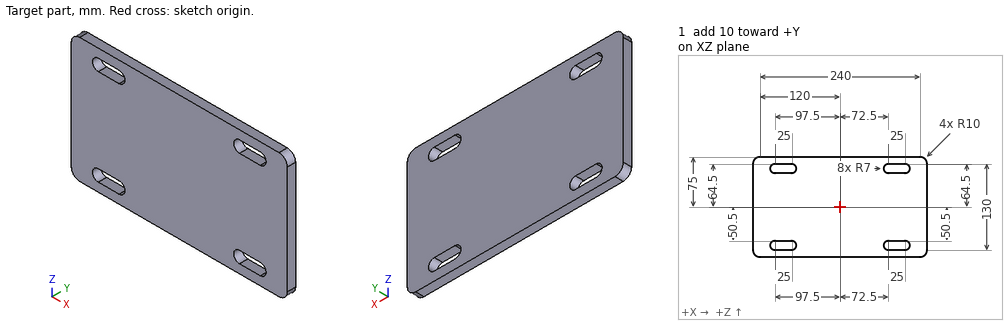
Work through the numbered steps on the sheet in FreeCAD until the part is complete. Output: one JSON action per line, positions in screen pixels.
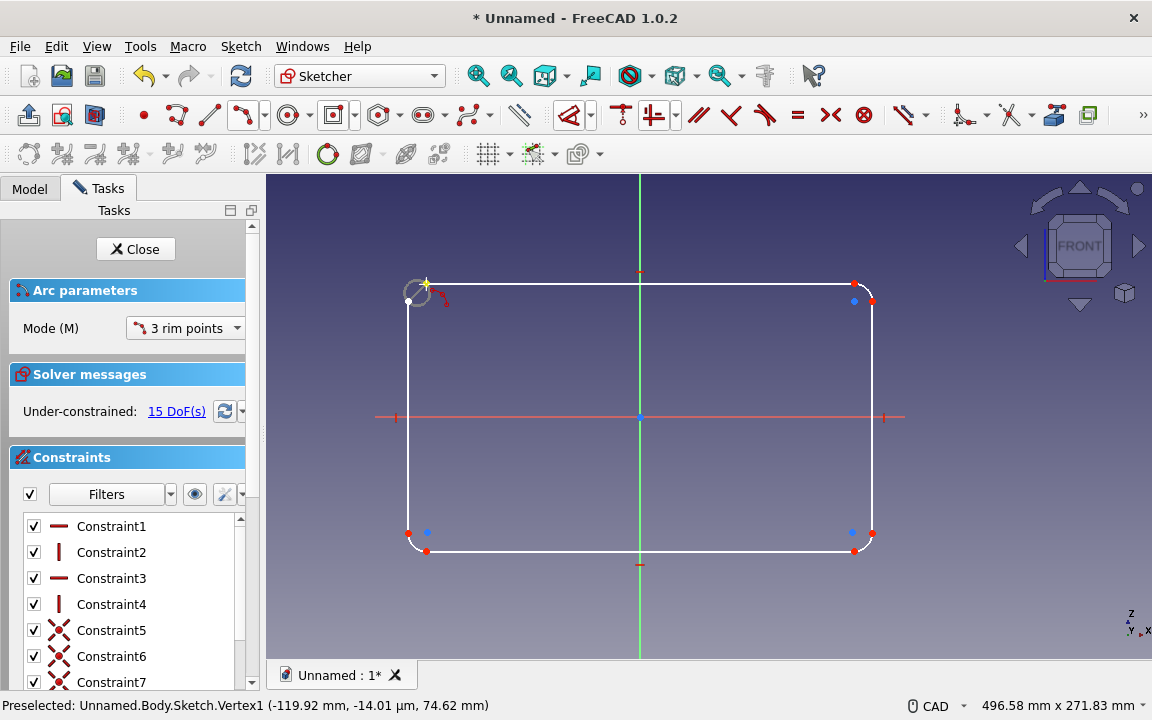
{"action": "scroll", "coordinate": [414, 289], "scroll_direction": "up", "scroll_amount": 6}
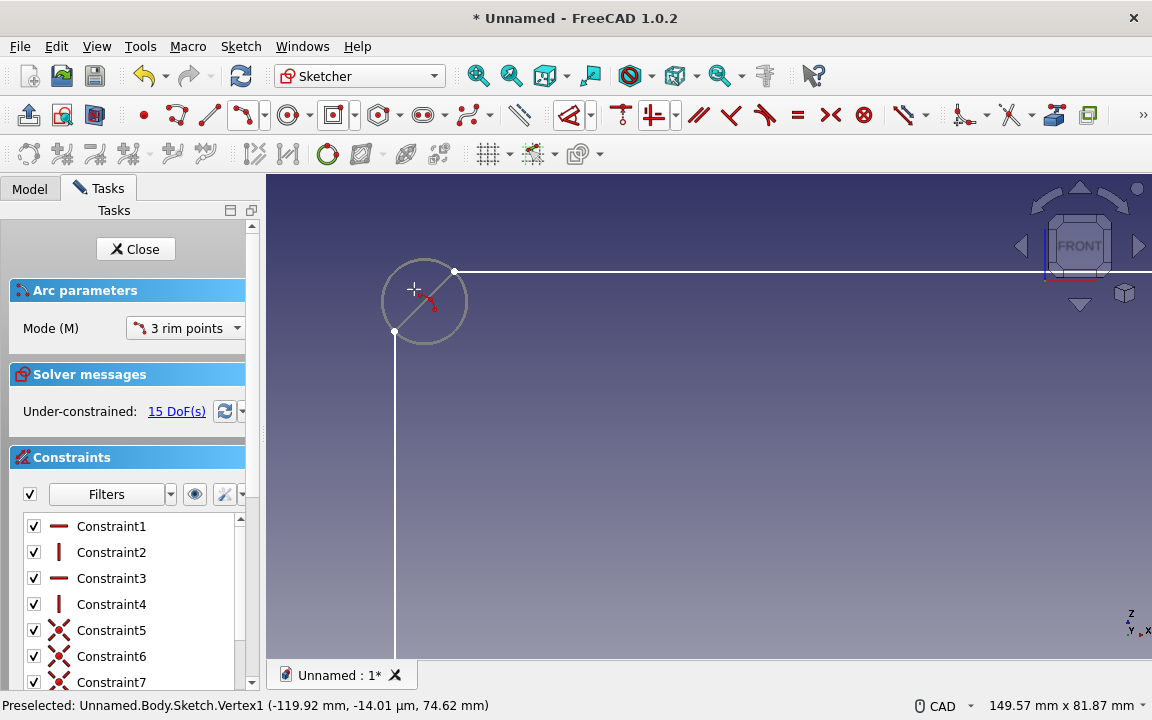
{"action": "left_click", "coordinate": [412, 287]}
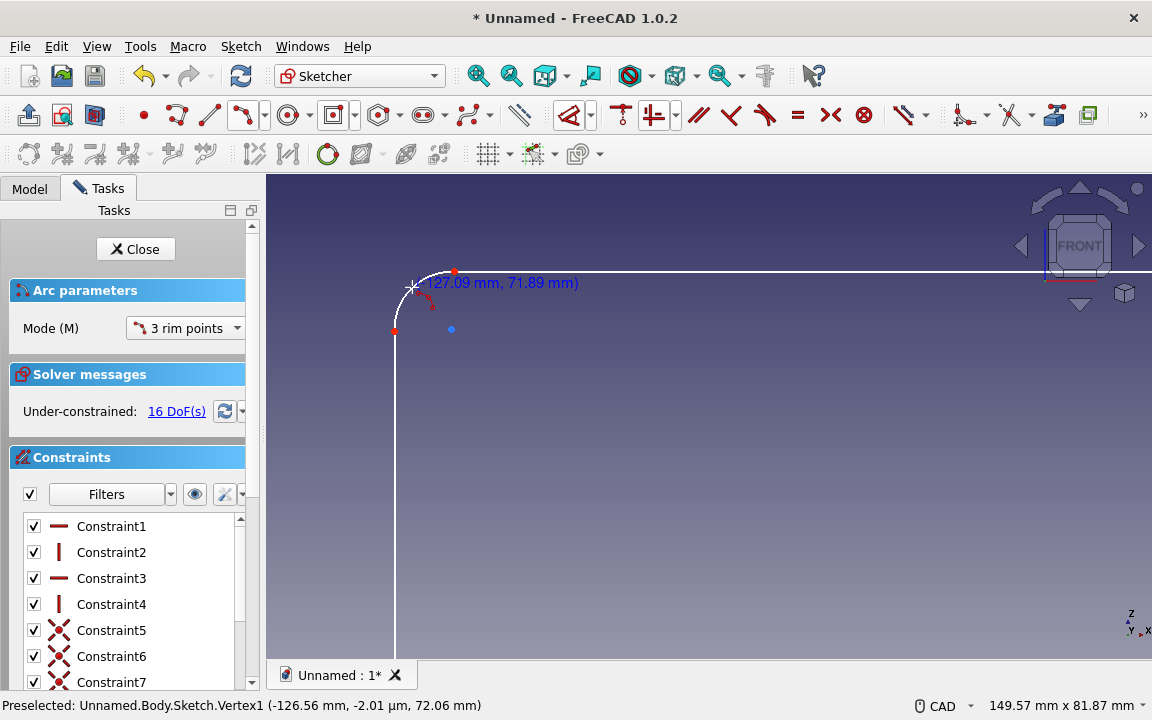
{"action": "left_click", "coordinate": [422, 116]}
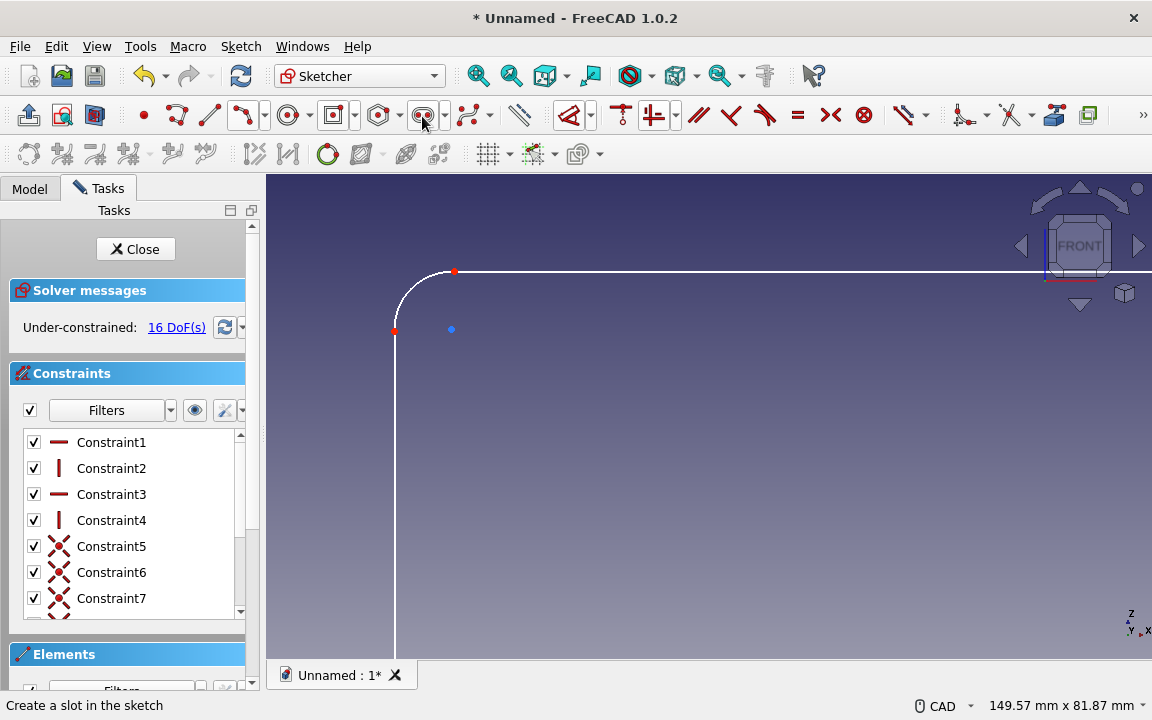
{"action": "scroll", "coordinate": [414, 288], "scroll_direction": "down", "scroll_amount": 6}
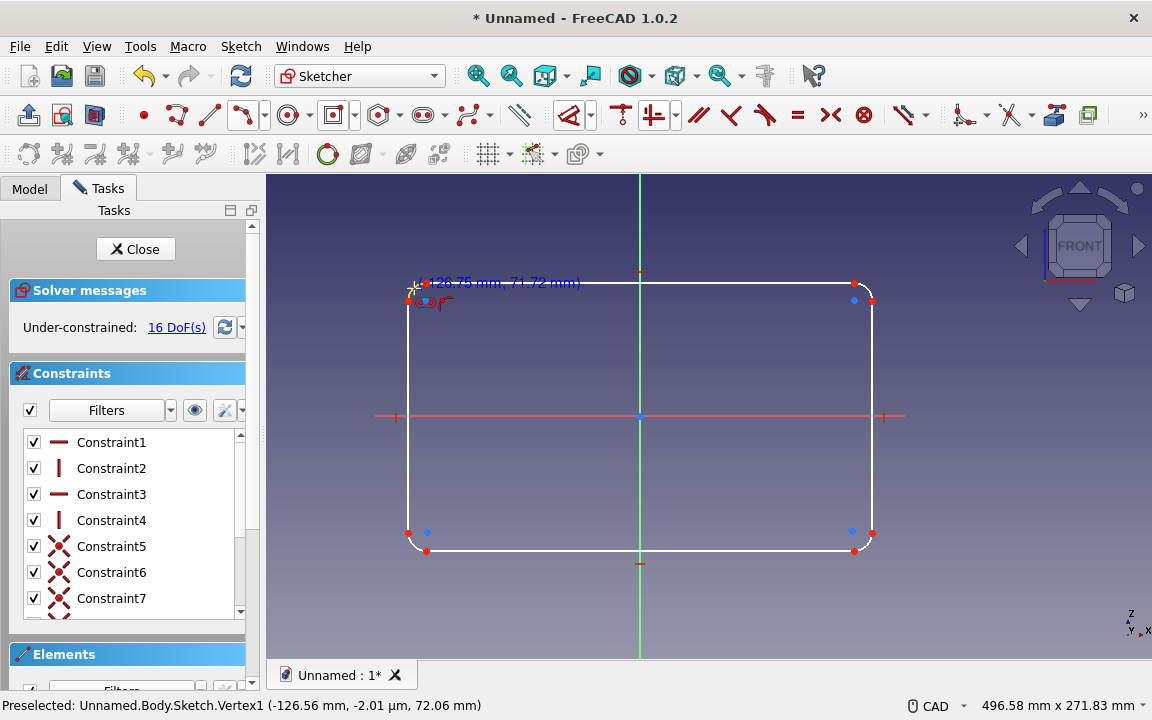
{"action": "scroll", "coordinate": [770, 314], "scroll_direction": "up", "scroll_amount": 3}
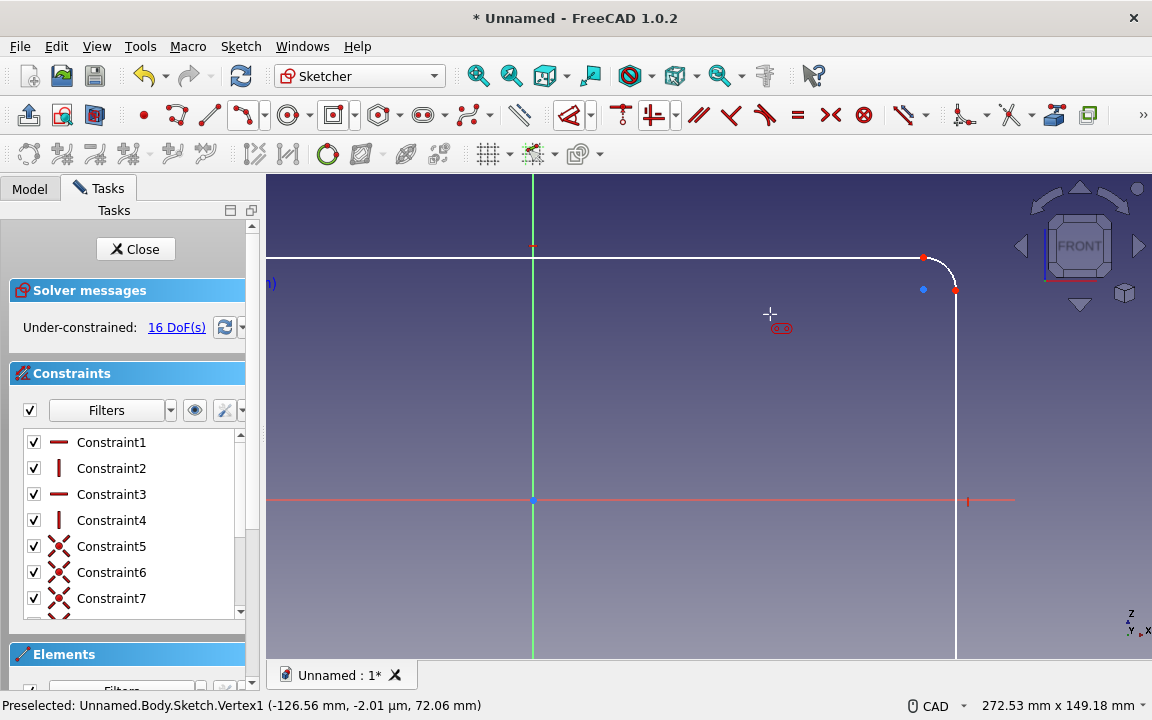
{"action": "left_click", "coordinate": [769, 313]}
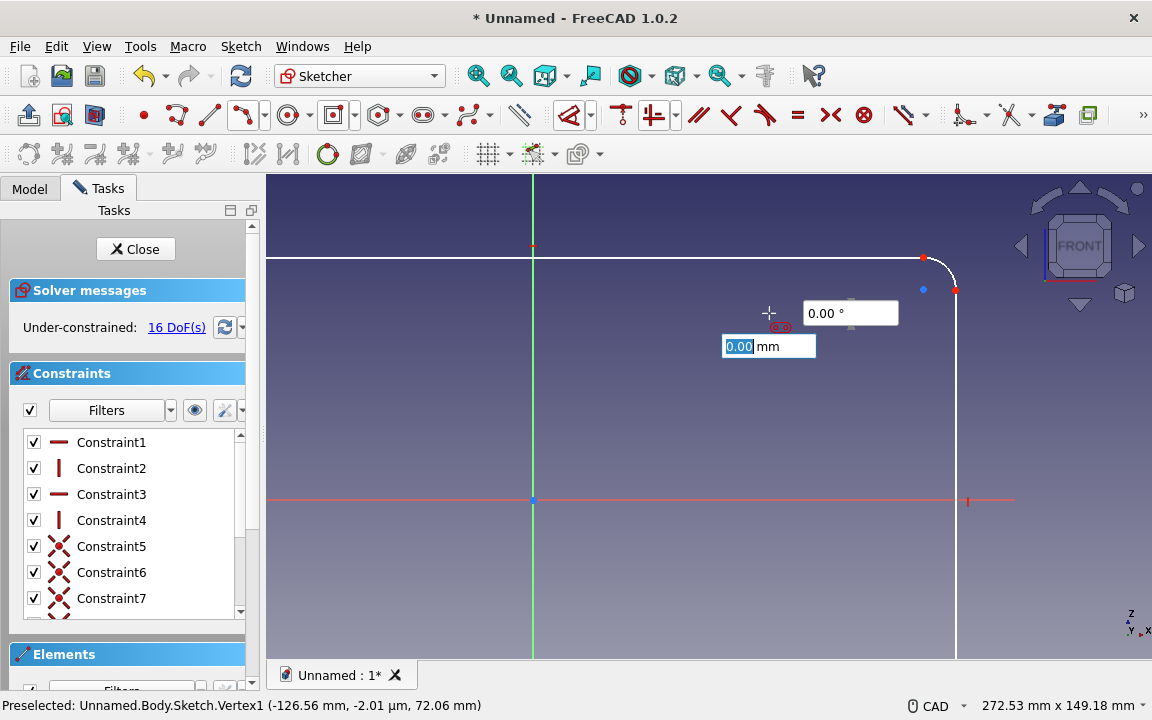
{"action": "left_click", "coordinate": [850, 313]}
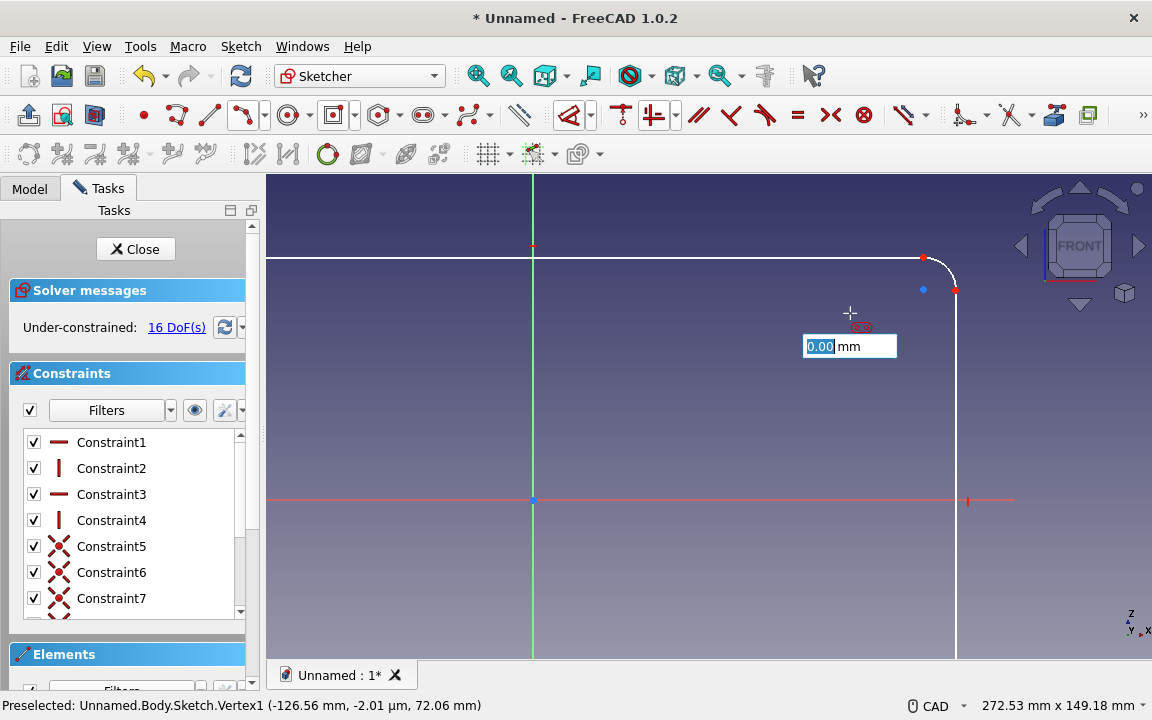
{"action": "left_click", "coordinate": [809, 336]}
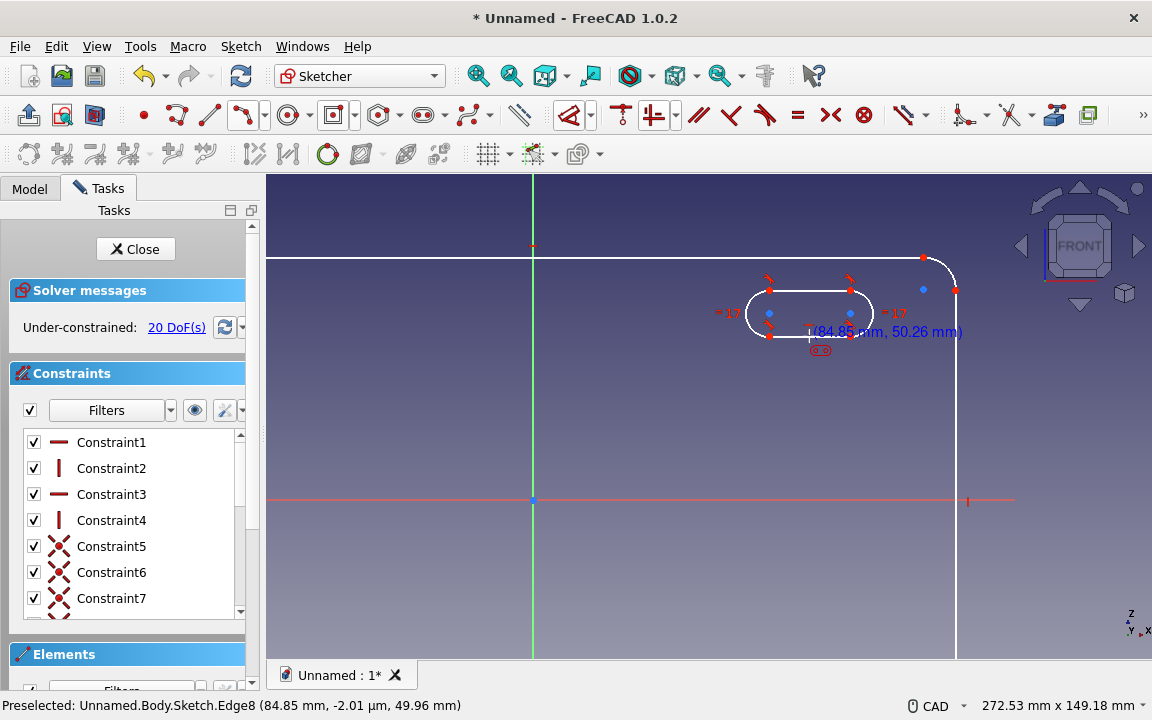
{"action": "scroll", "coordinate": [771, 314], "scroll_direction": "down", "scroll_amount": 3}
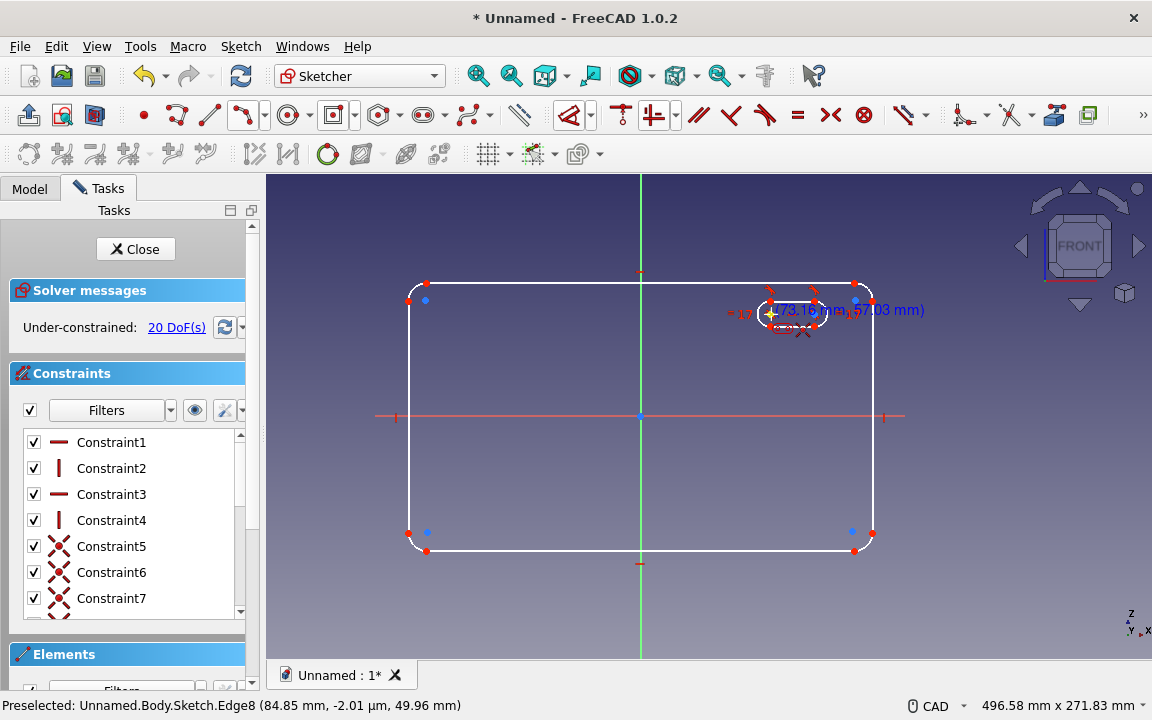
{"action": "scroll", "coordinate": [467, 314], "scroll_direction": "up", "scroll_amount": 3}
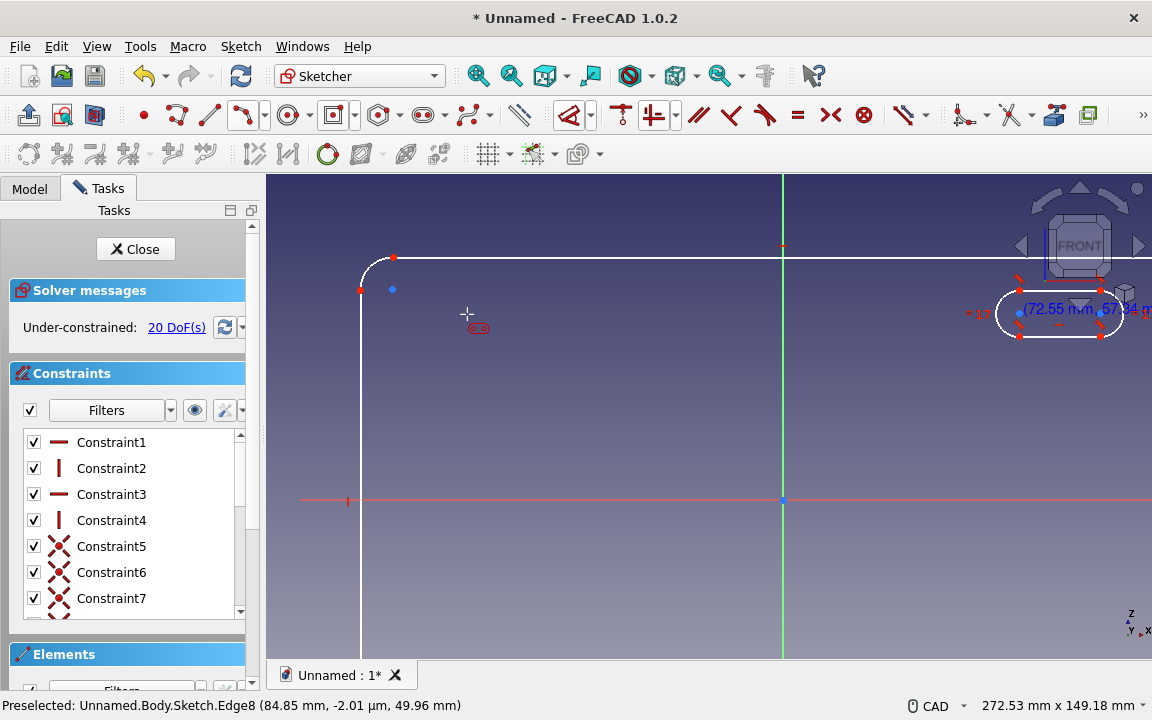
{"action": "left_click", "coordinate": [466, 313]}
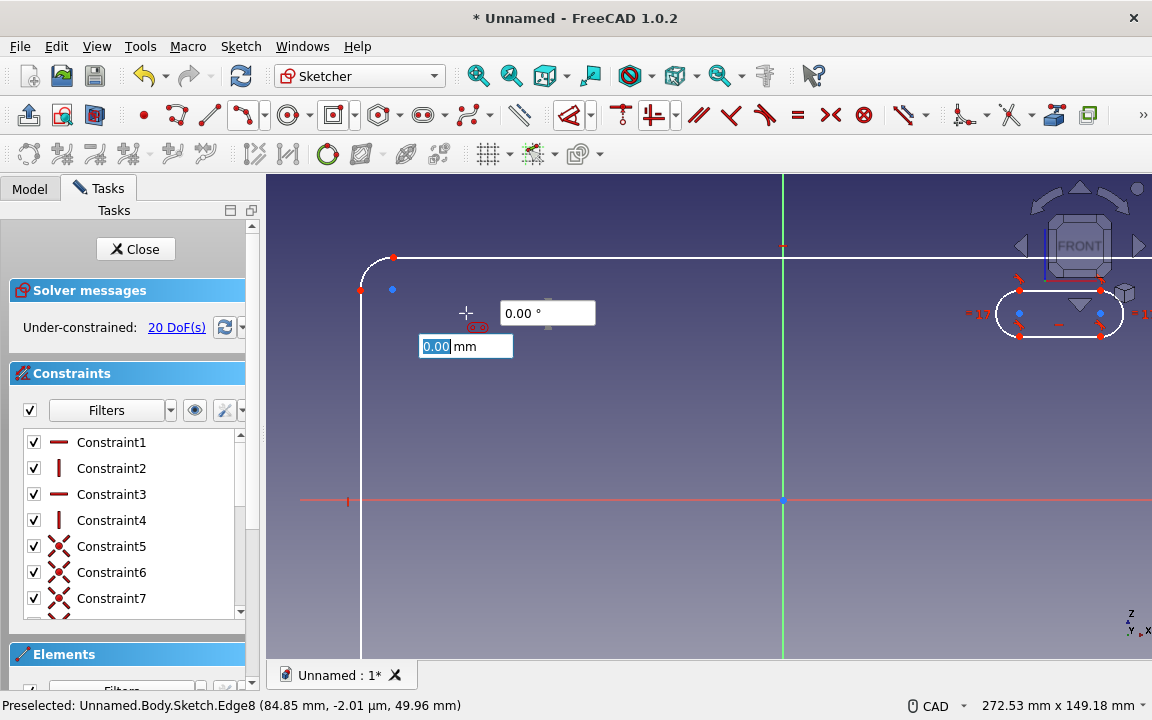
{"action": "left_click", "coordinate": [548, 313]}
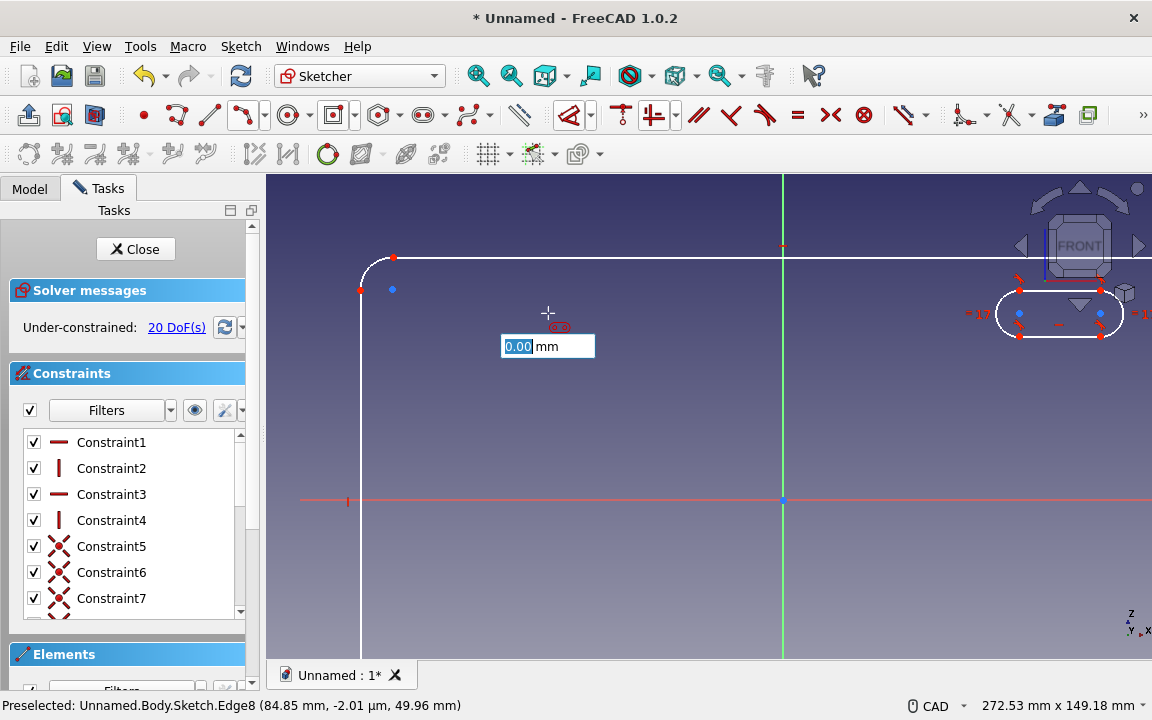
{"action": "left_click", "coordinate": [507, 291]}